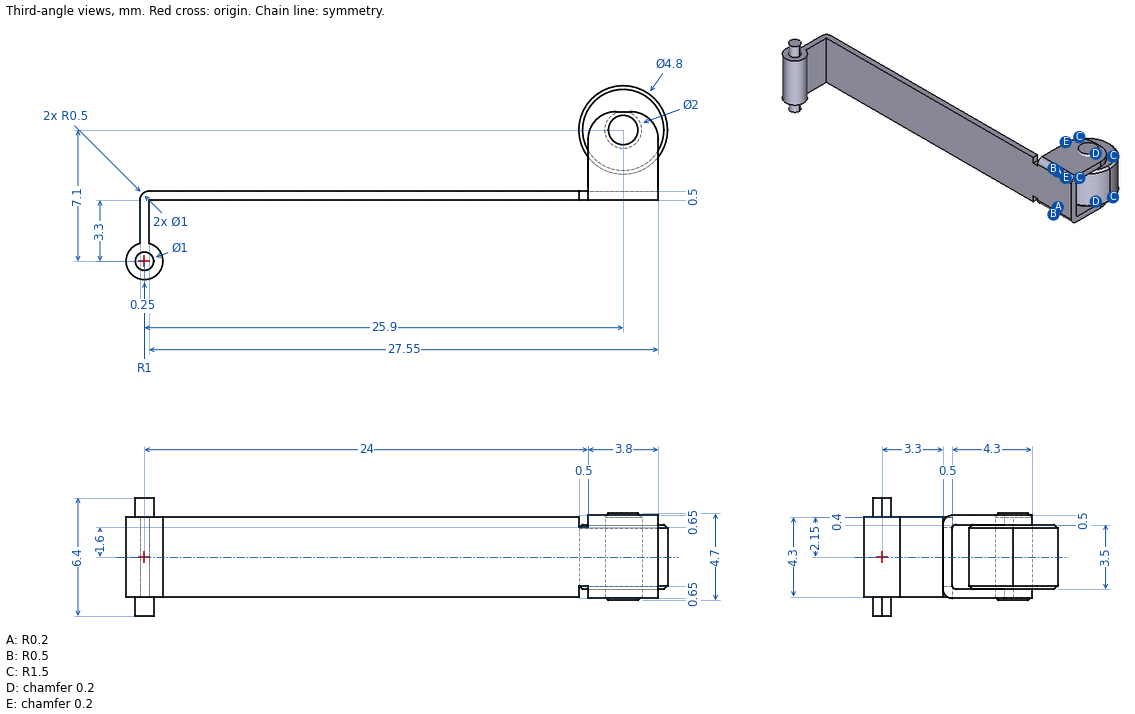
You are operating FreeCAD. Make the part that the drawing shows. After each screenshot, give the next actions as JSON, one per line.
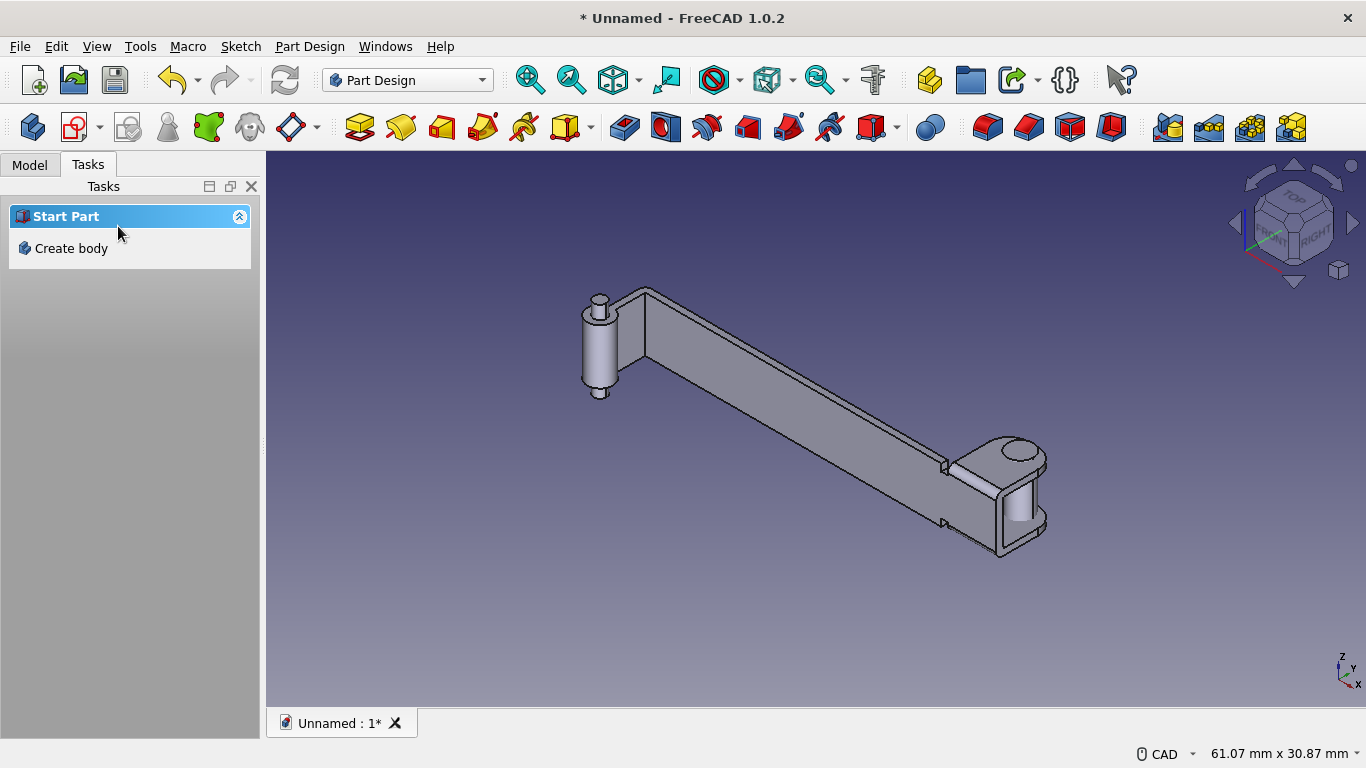
{"action": "key", "text": "v f"}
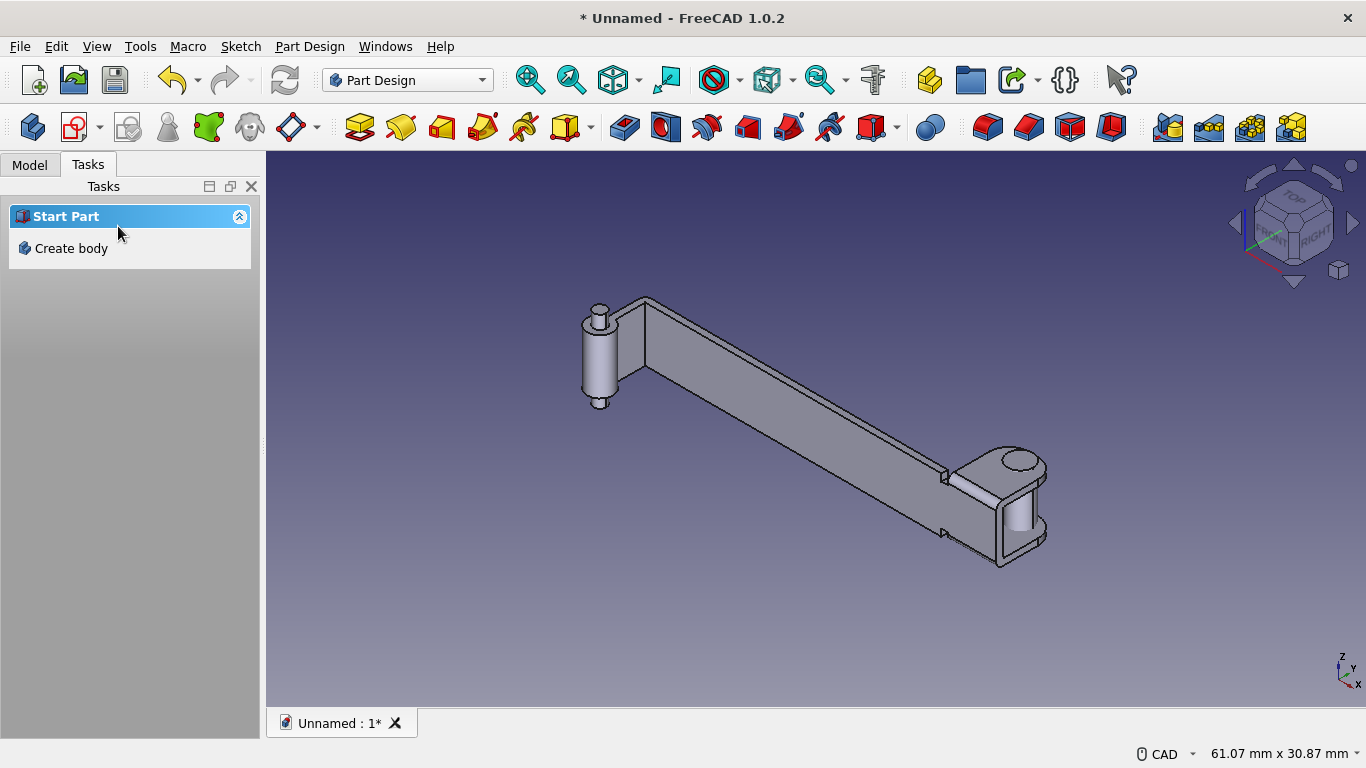
{"action": "left_click", "coordinate": [1008, 452]}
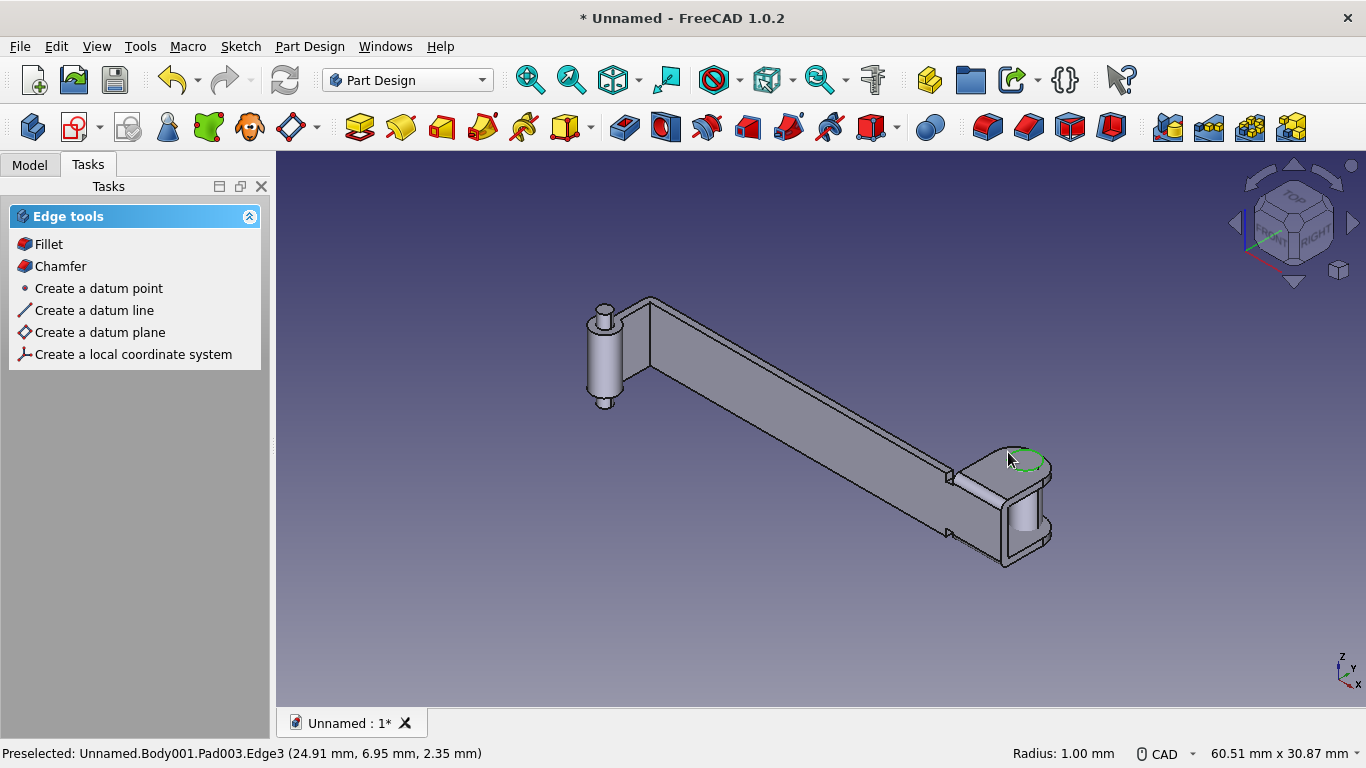
{"action": "key", "text": "2"}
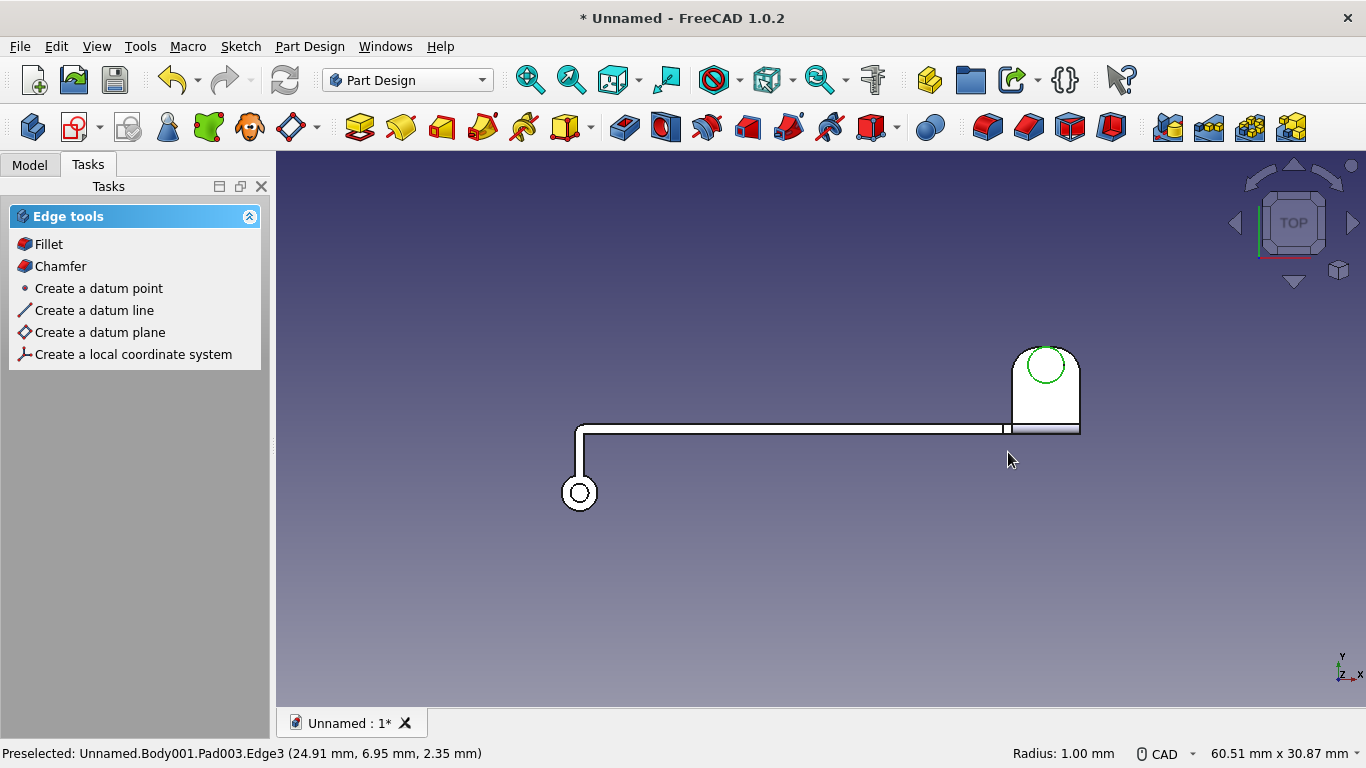
{"action": "key", "text": "v f"}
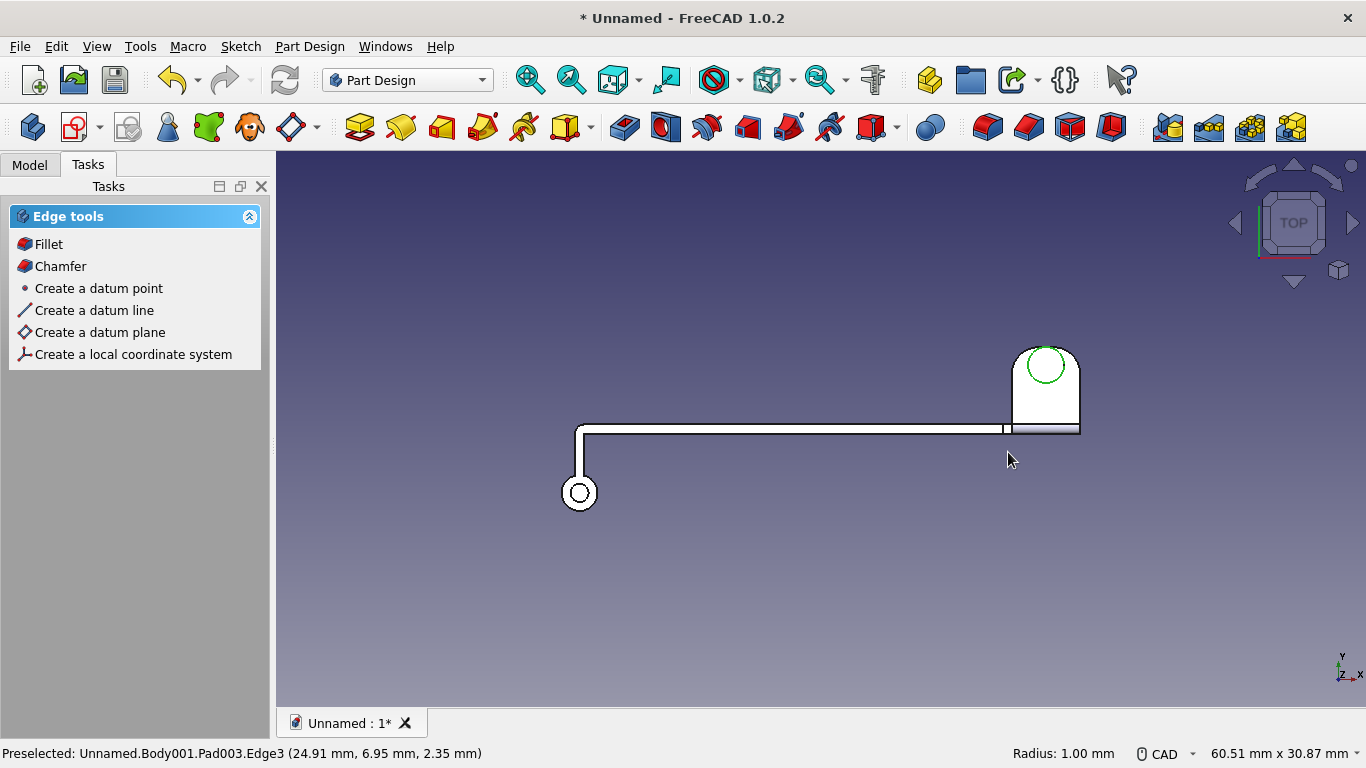
{"action": "key", "text": "0"}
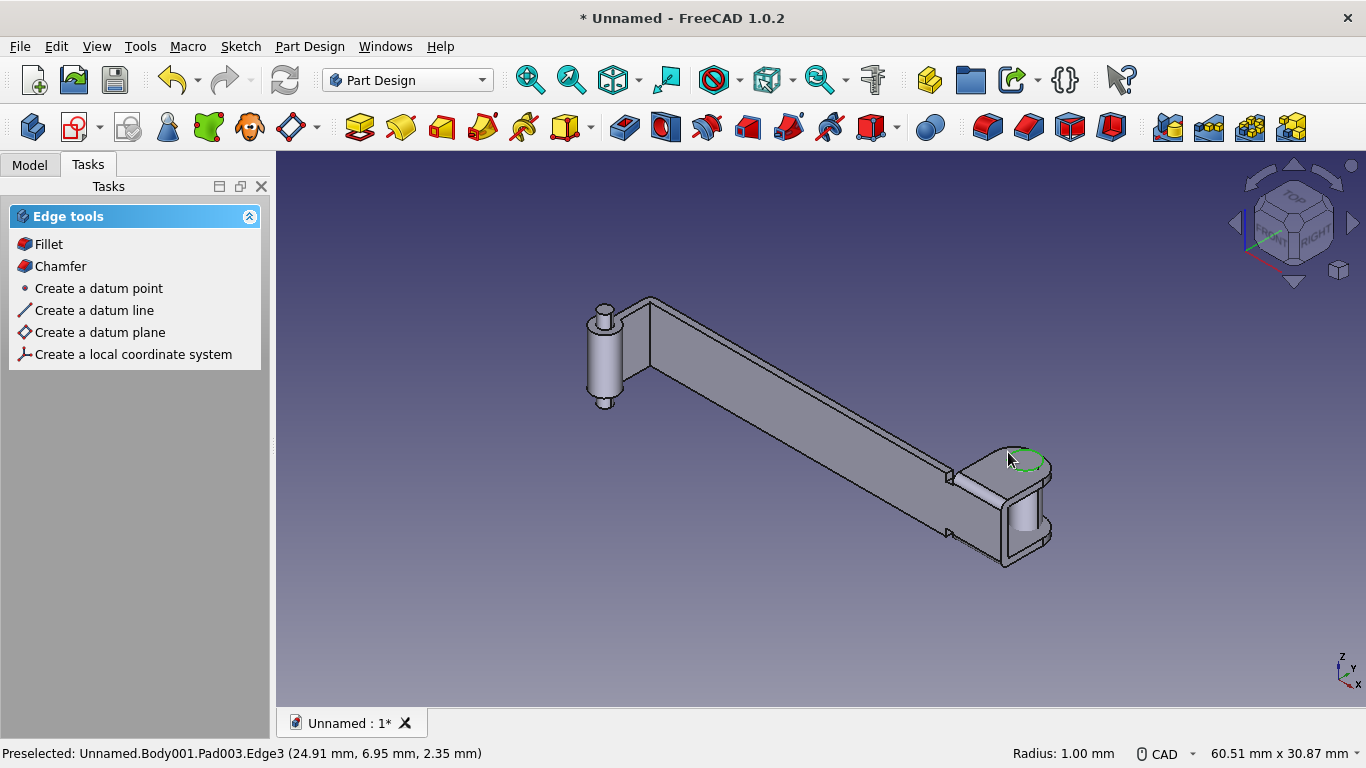
{"action": "left_click", "coordinate": [531, 80]}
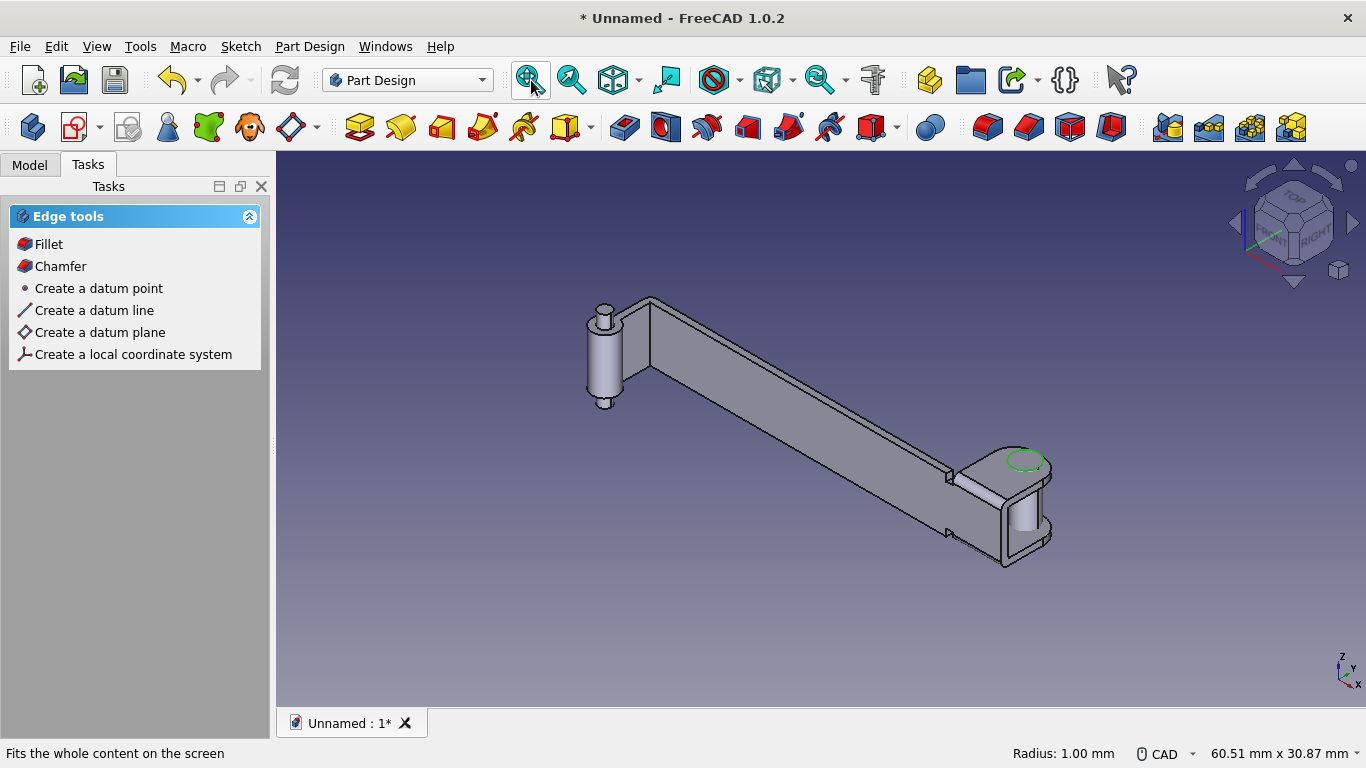
{"action": "key", "text": "1"}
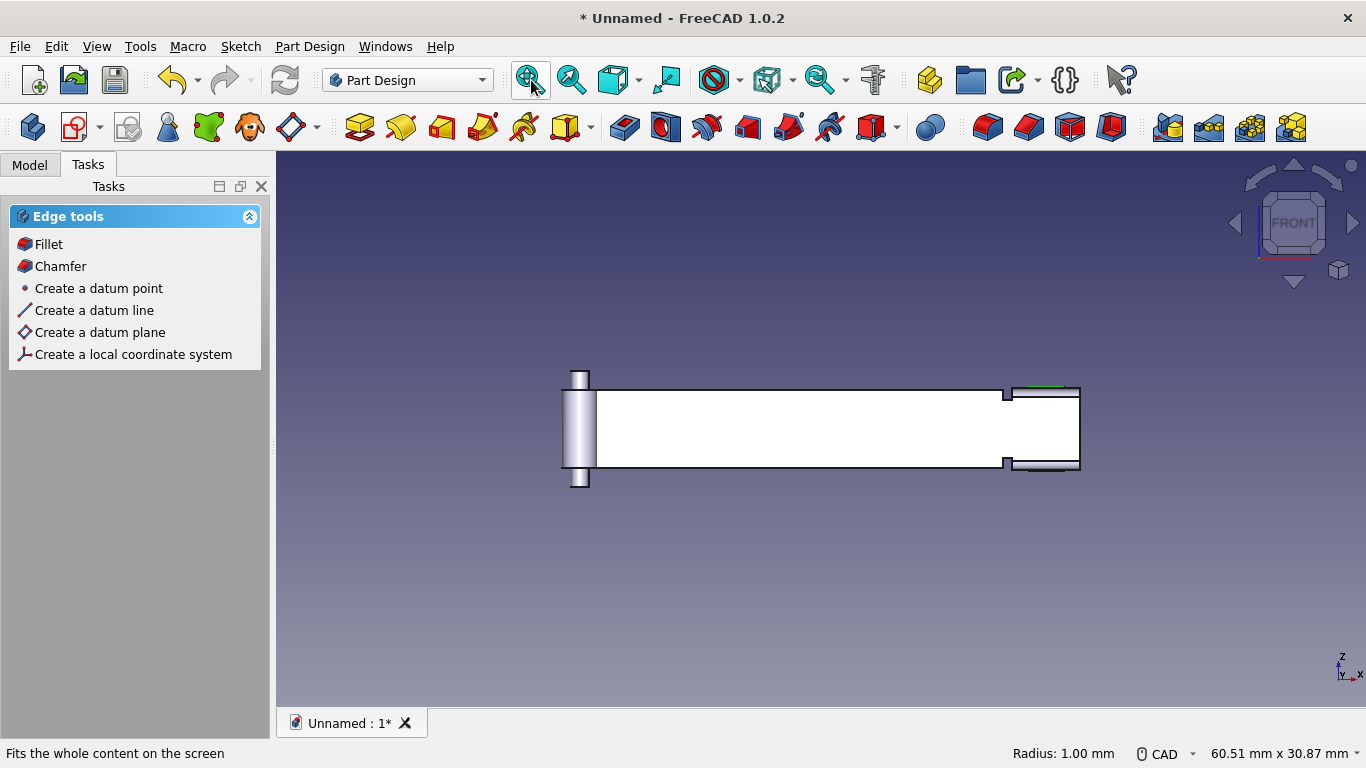
{"action": "key", "text": "v f"}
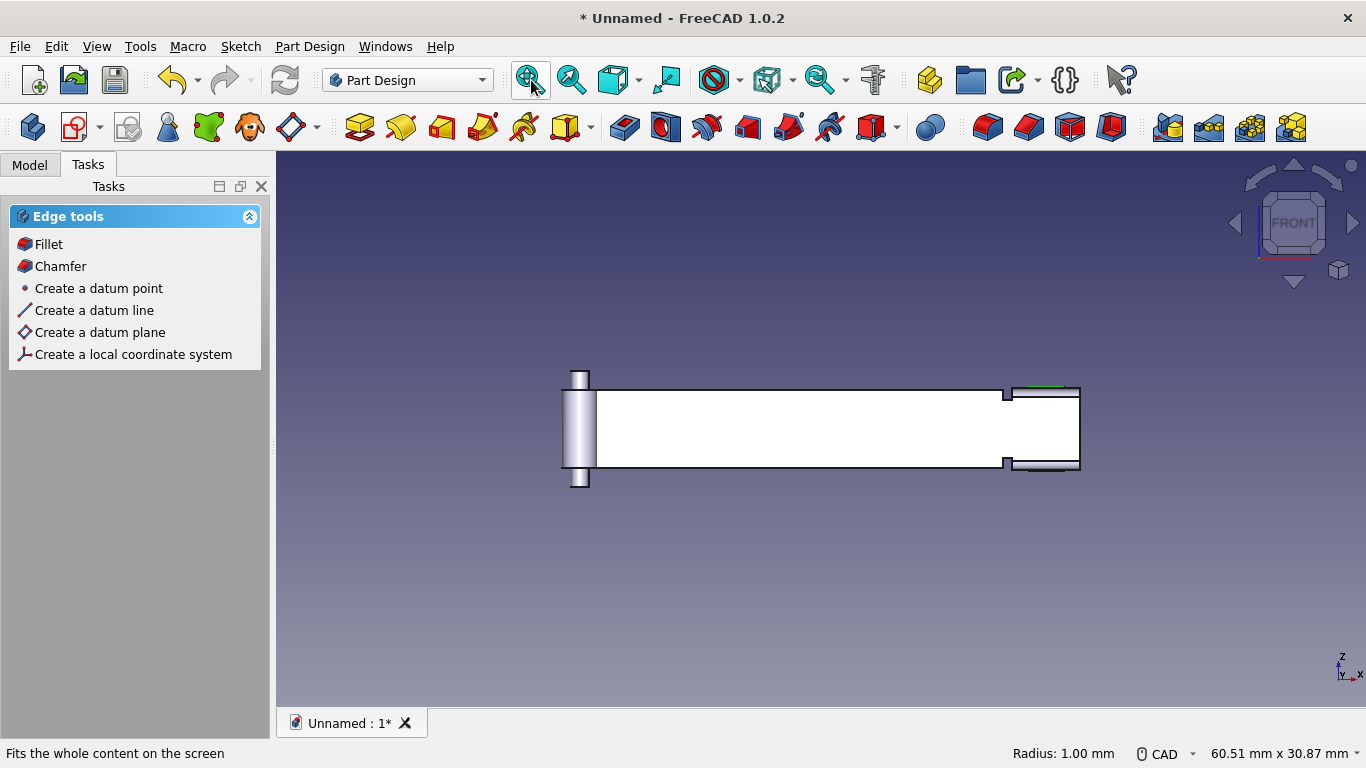
{"action": "key", "text": "3"}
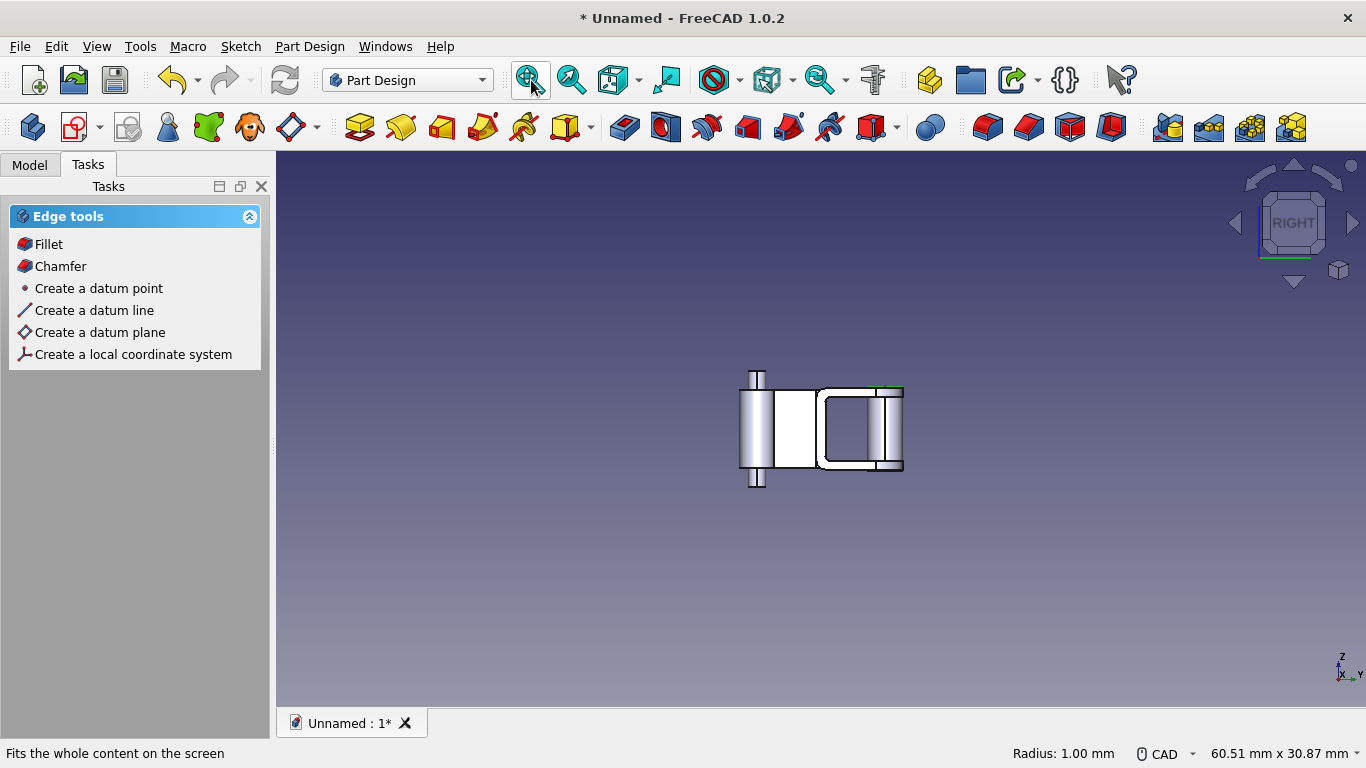
{"action": "key", "text": "v f"}